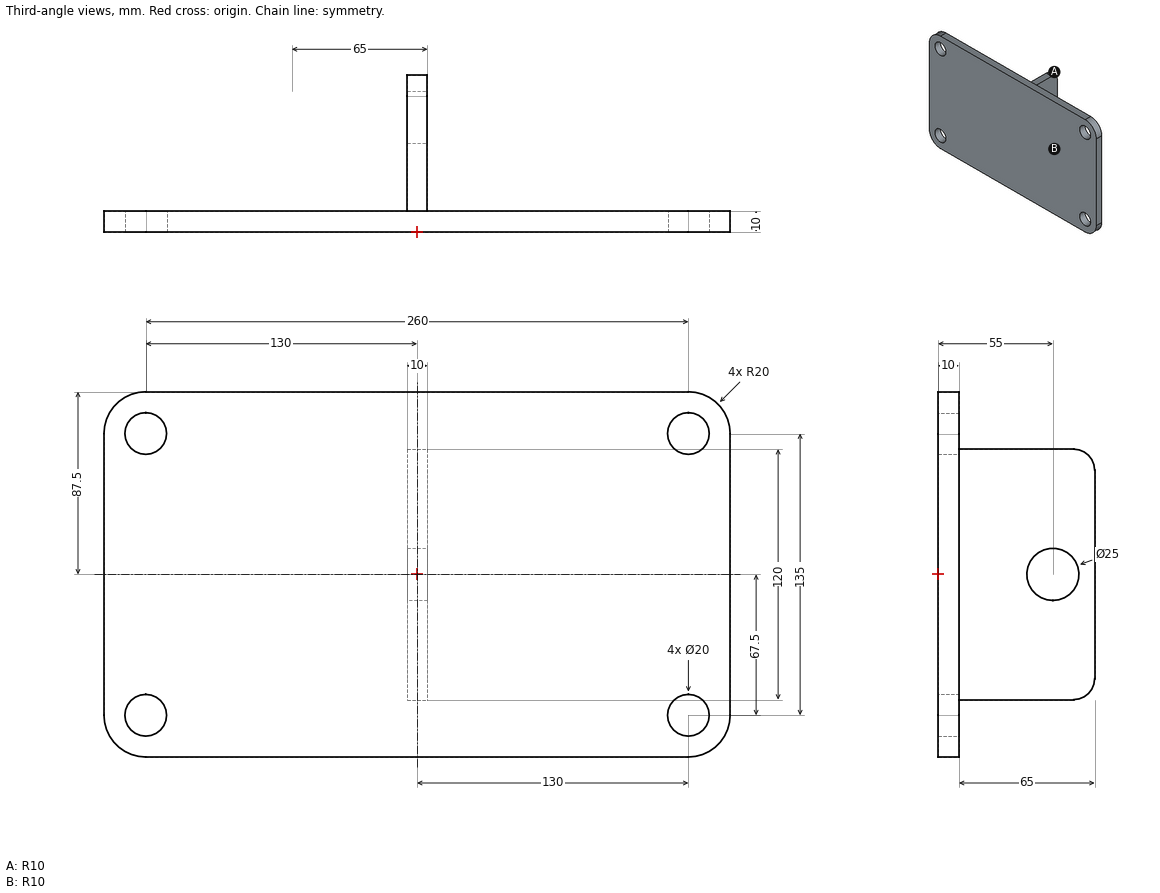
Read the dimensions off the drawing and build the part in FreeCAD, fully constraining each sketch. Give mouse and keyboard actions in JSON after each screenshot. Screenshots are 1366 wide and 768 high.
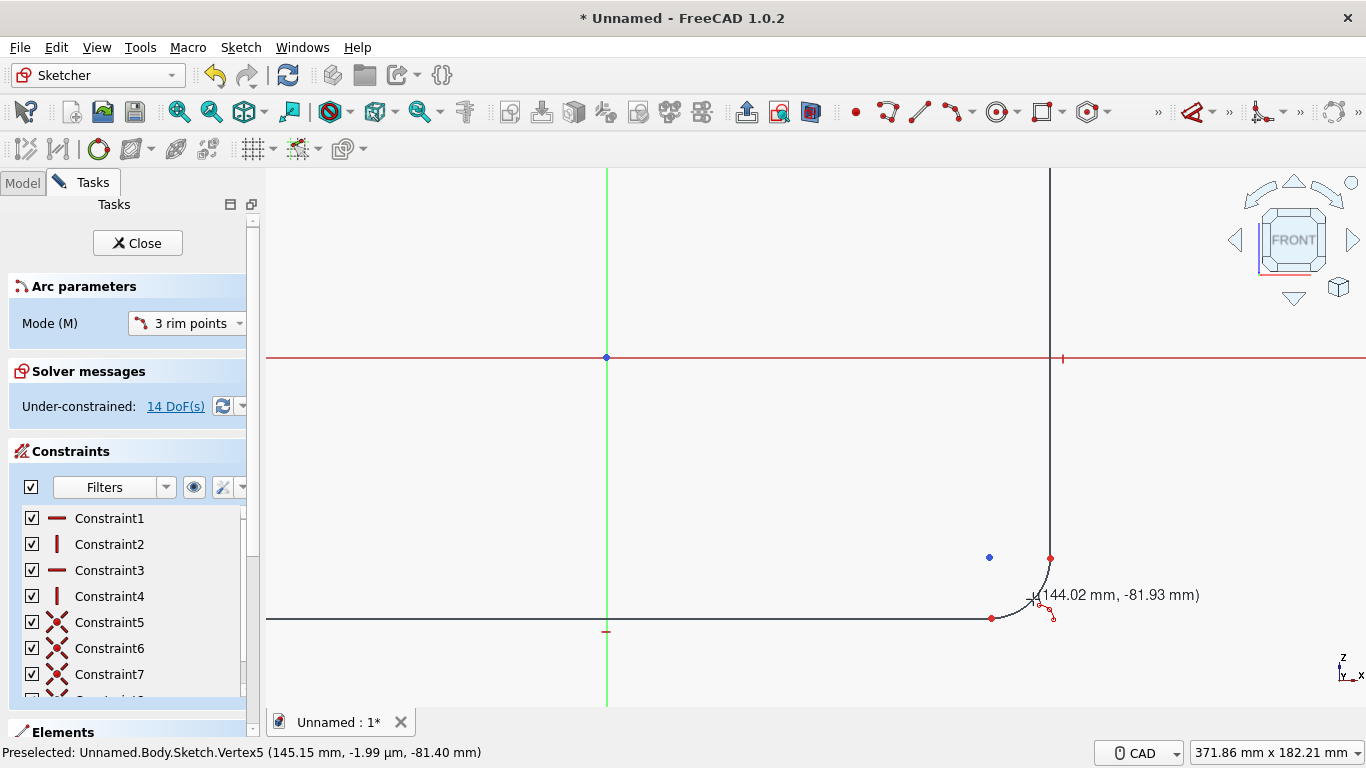
{"action": "scroll", "coordinate": [1033, 600], "scroll_direction": "down", "scroll_amount": 2}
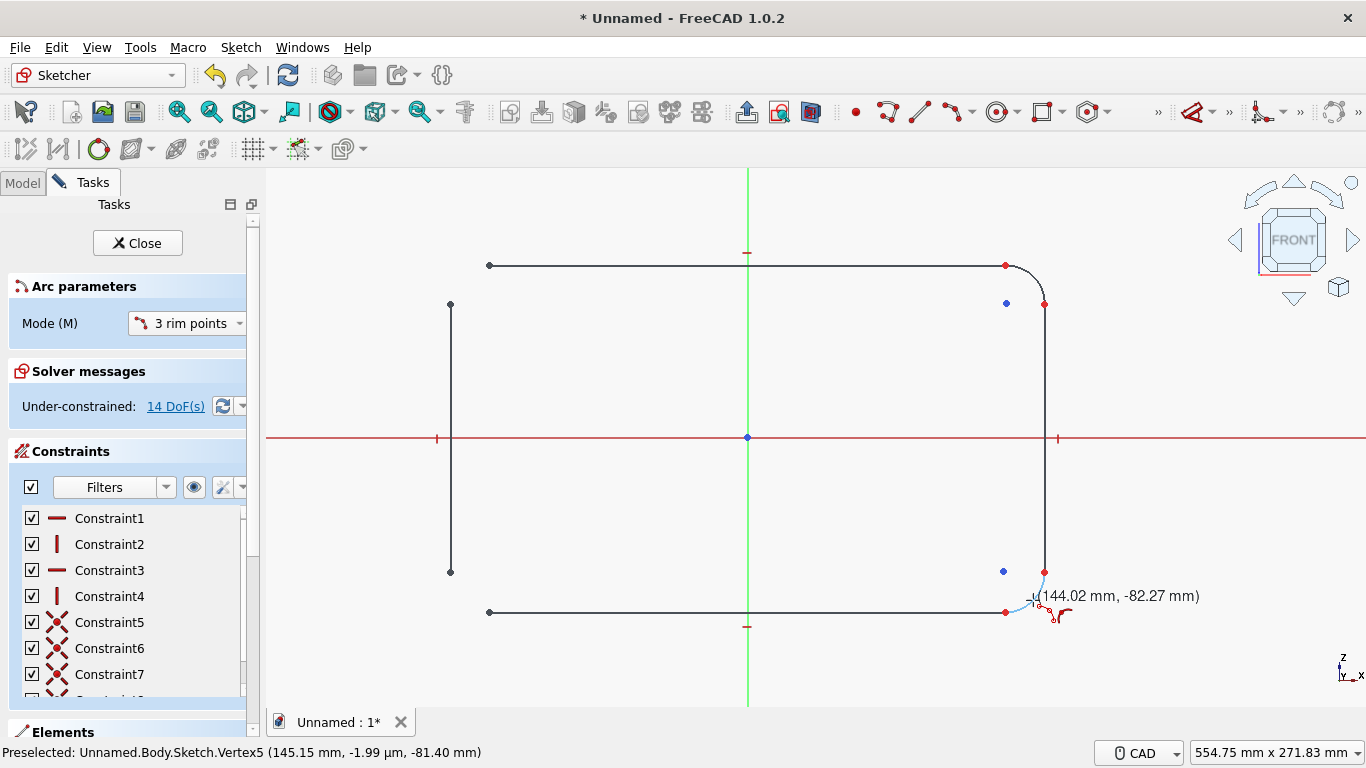
{"action": "left_click", "coordinate": [490, 613]}
{"action": "left_click", "coordinate": [451, 573]}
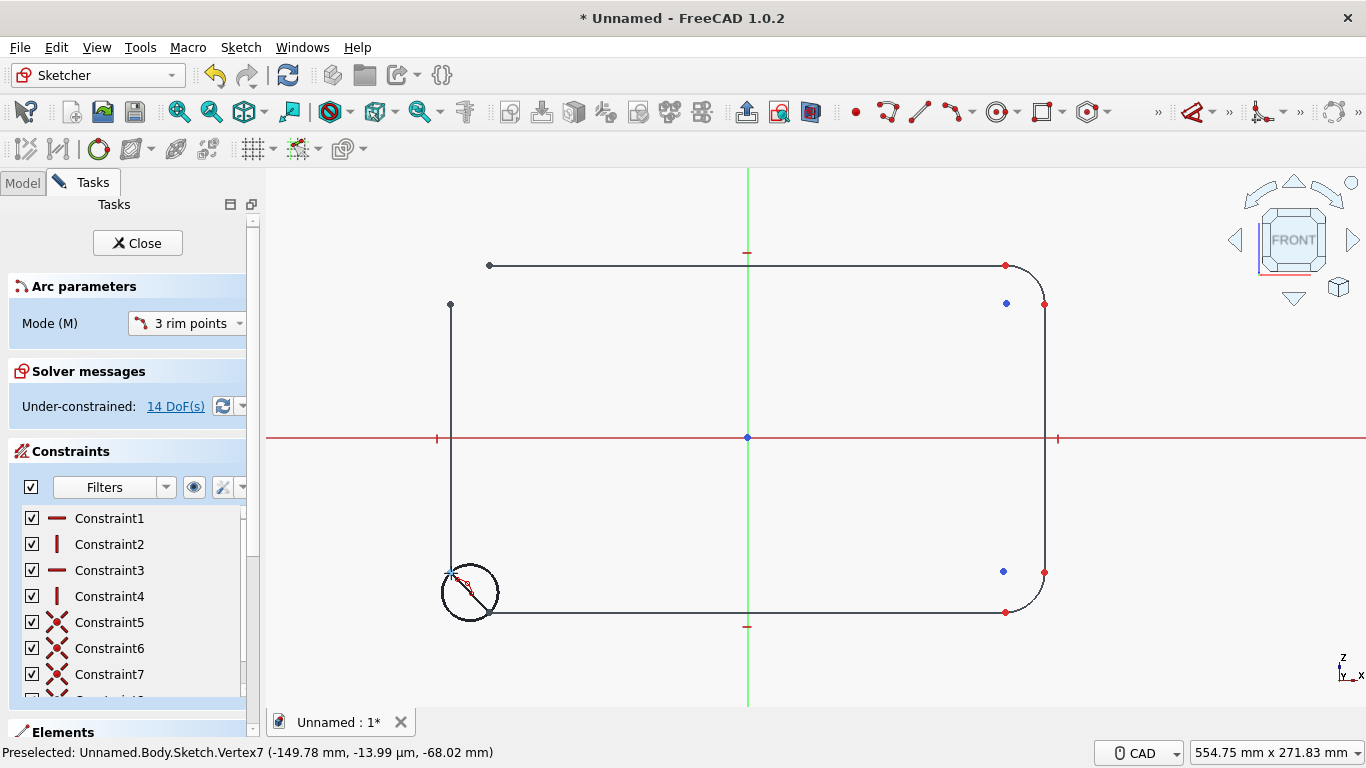
{"action": "scroll", "coordinate": [462, 600], "scroll_direction": "up", "scroll_amount": 2}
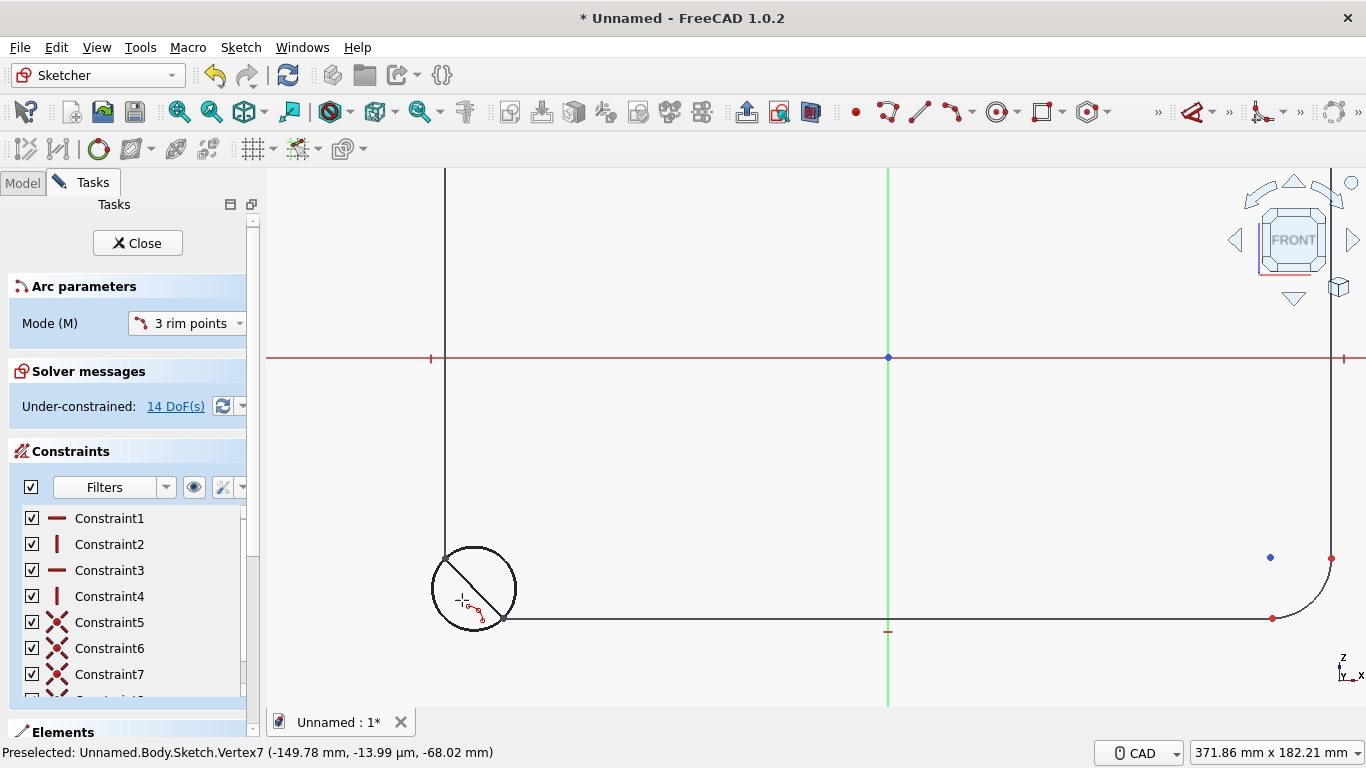
{"action": "left_click", "coordinate": [462, 599]}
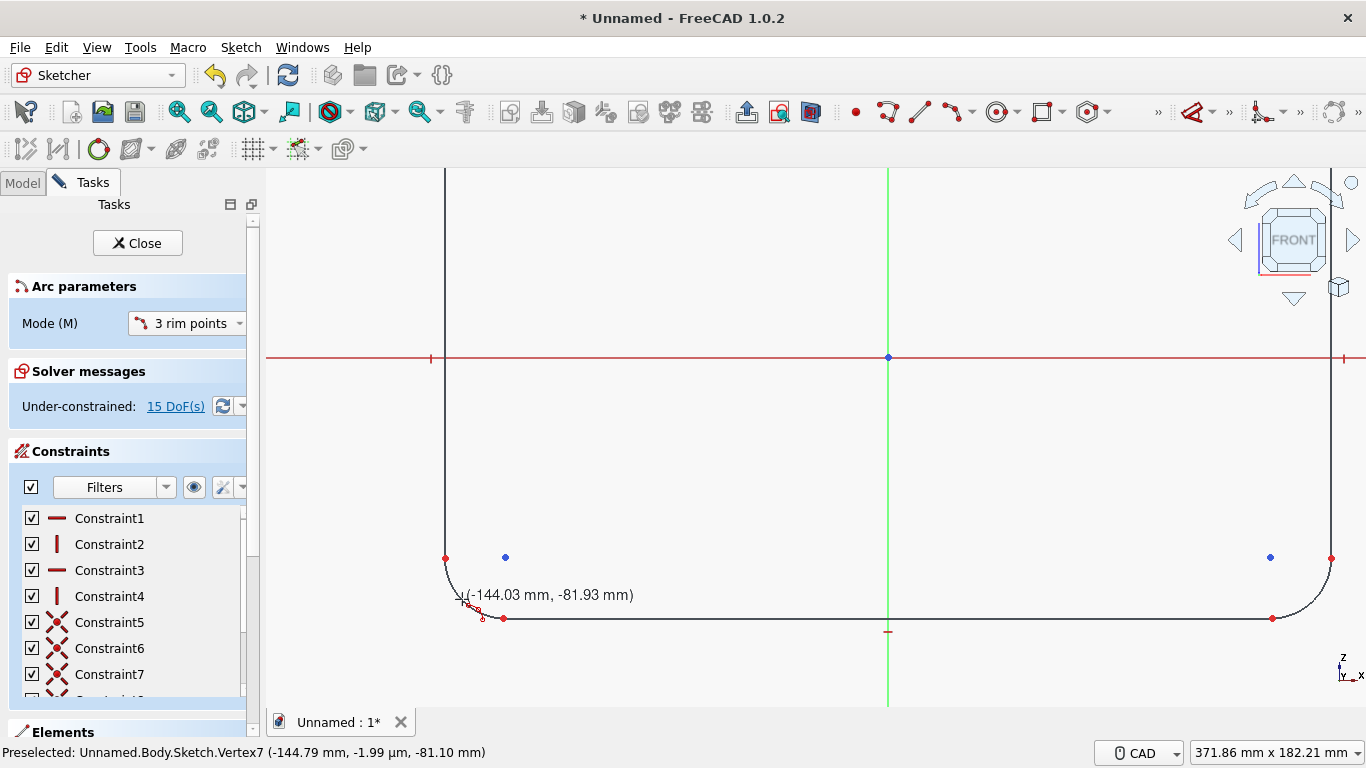
{"action": "scroll", "coordinate": [462, 600], "scroll_direction": "down", "scroll_amount": 2}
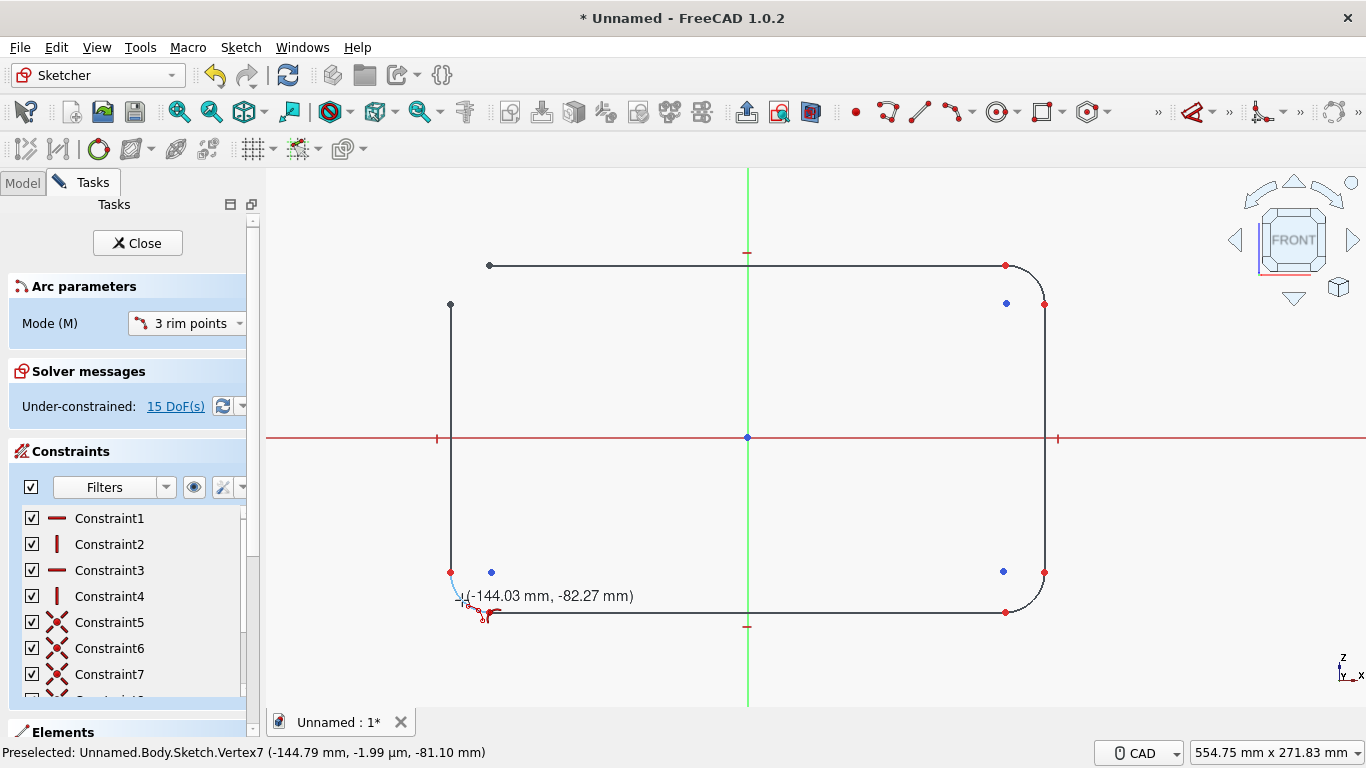
{"action": "left_click", "coordinate": [451, 305]}
{"action": "left_click", "coordinate": [490, 266]}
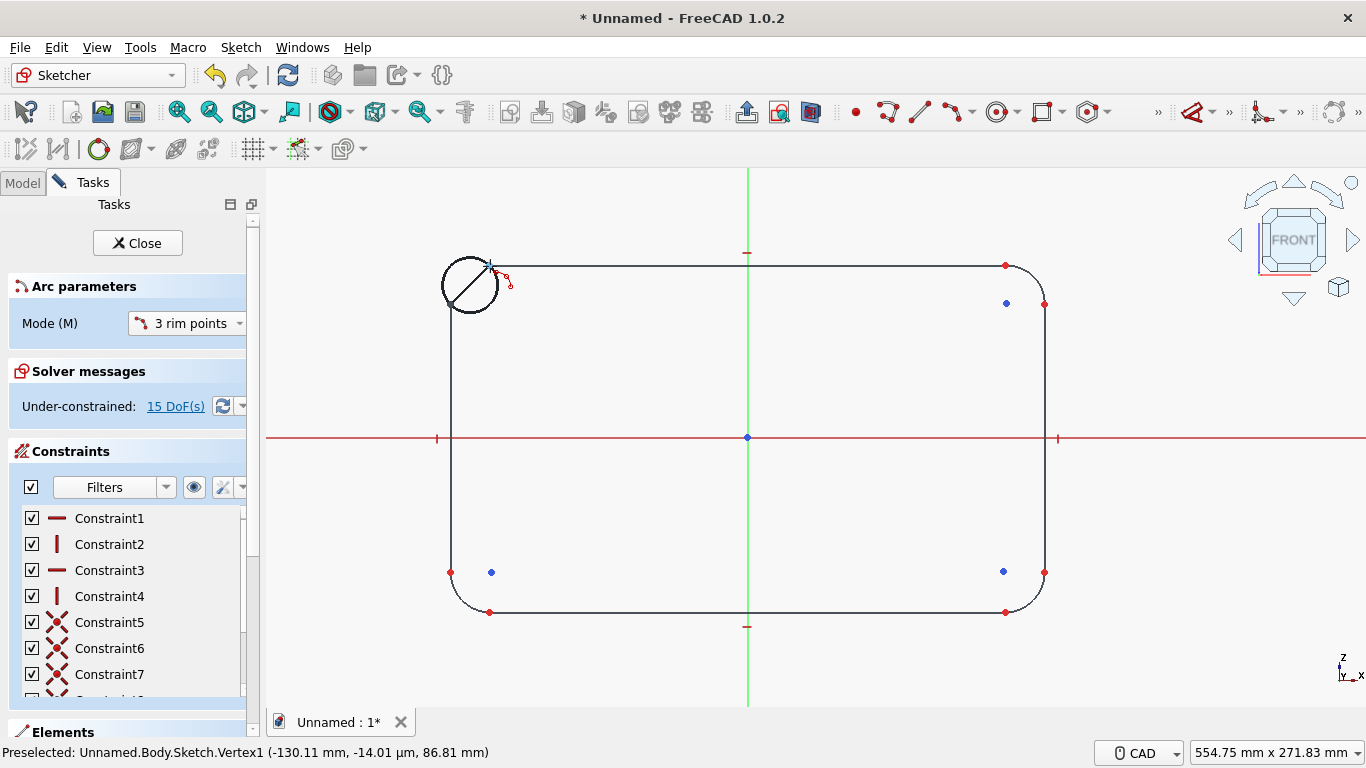
{"action": "scroll", "coordinate": [462, 276], "scroll_direction": "up", "scroll_amount": 2}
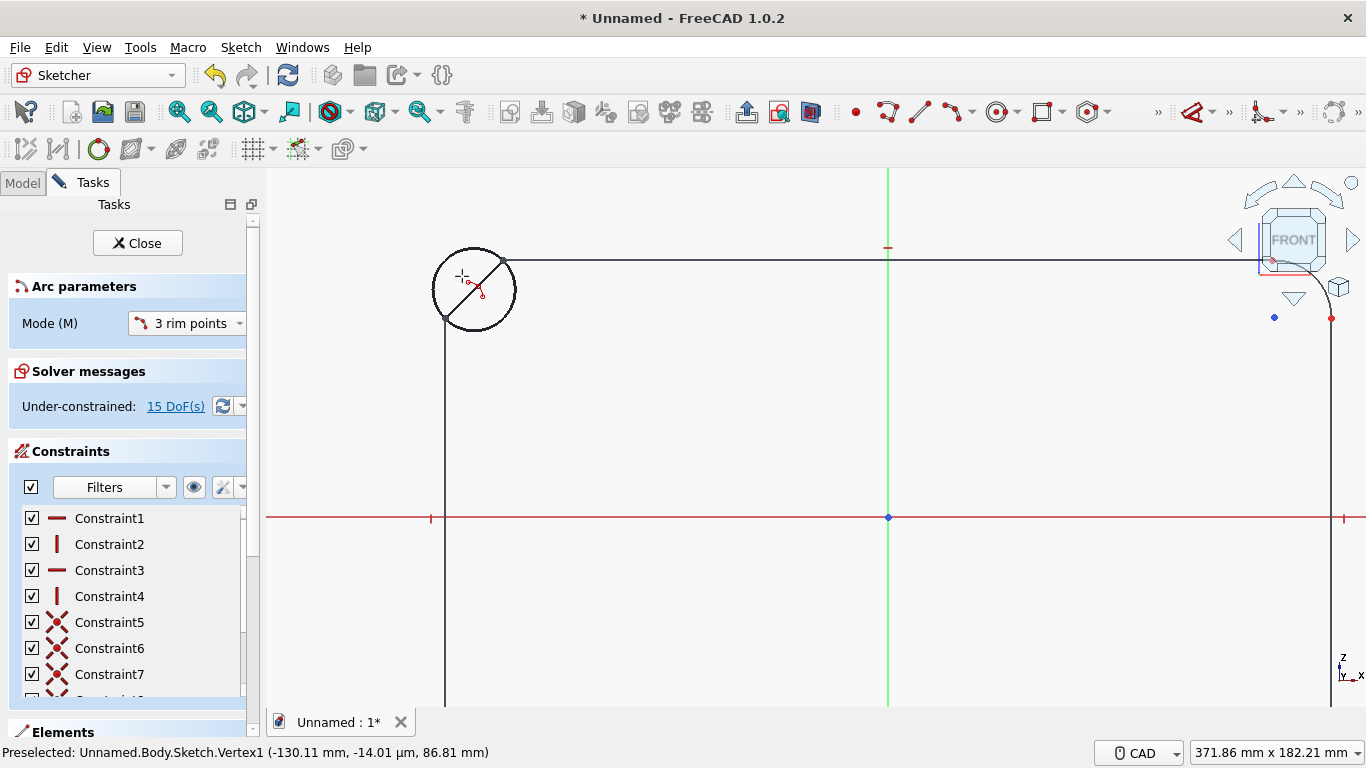
{"action": "left_click", "coordinate": [462, 276]}
{"action": "key", "text": "Escape"}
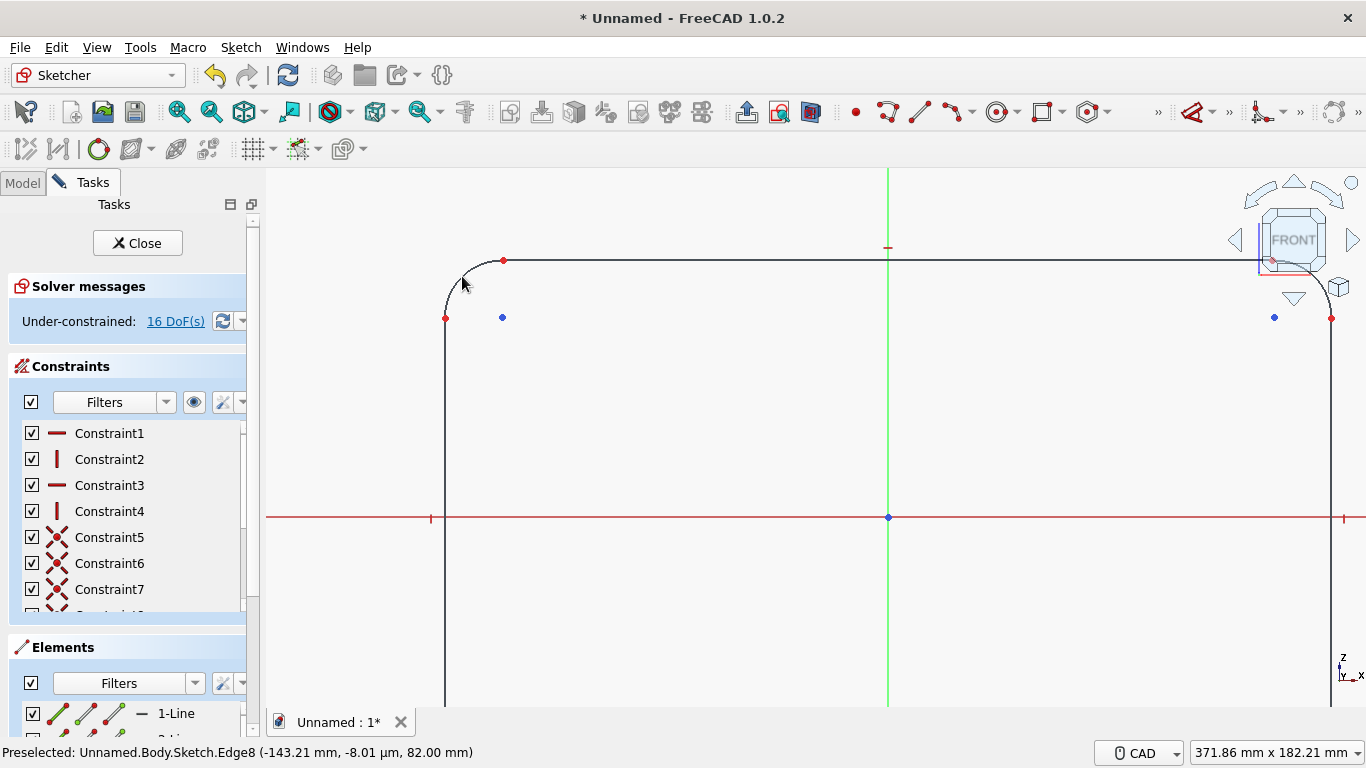
{"action": "left_click", "coordinate": [734, 260]}